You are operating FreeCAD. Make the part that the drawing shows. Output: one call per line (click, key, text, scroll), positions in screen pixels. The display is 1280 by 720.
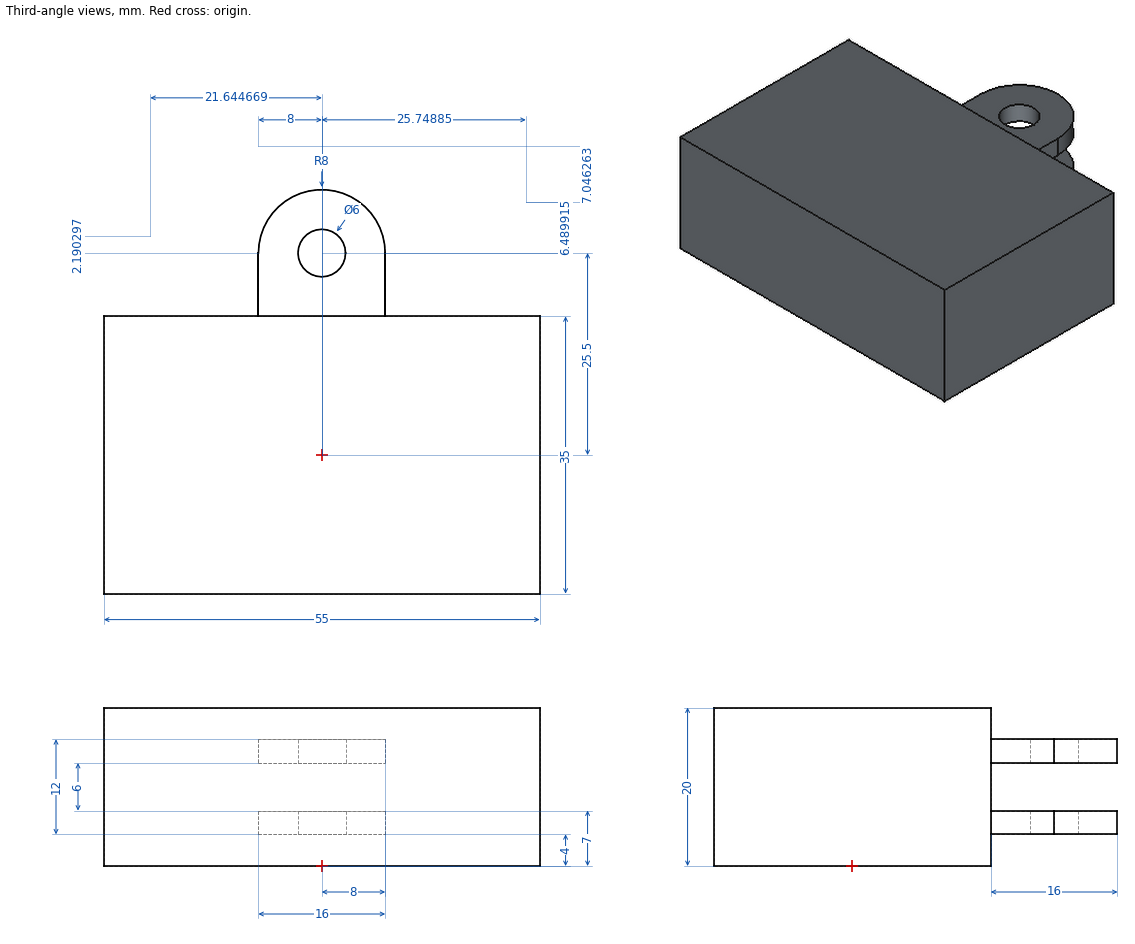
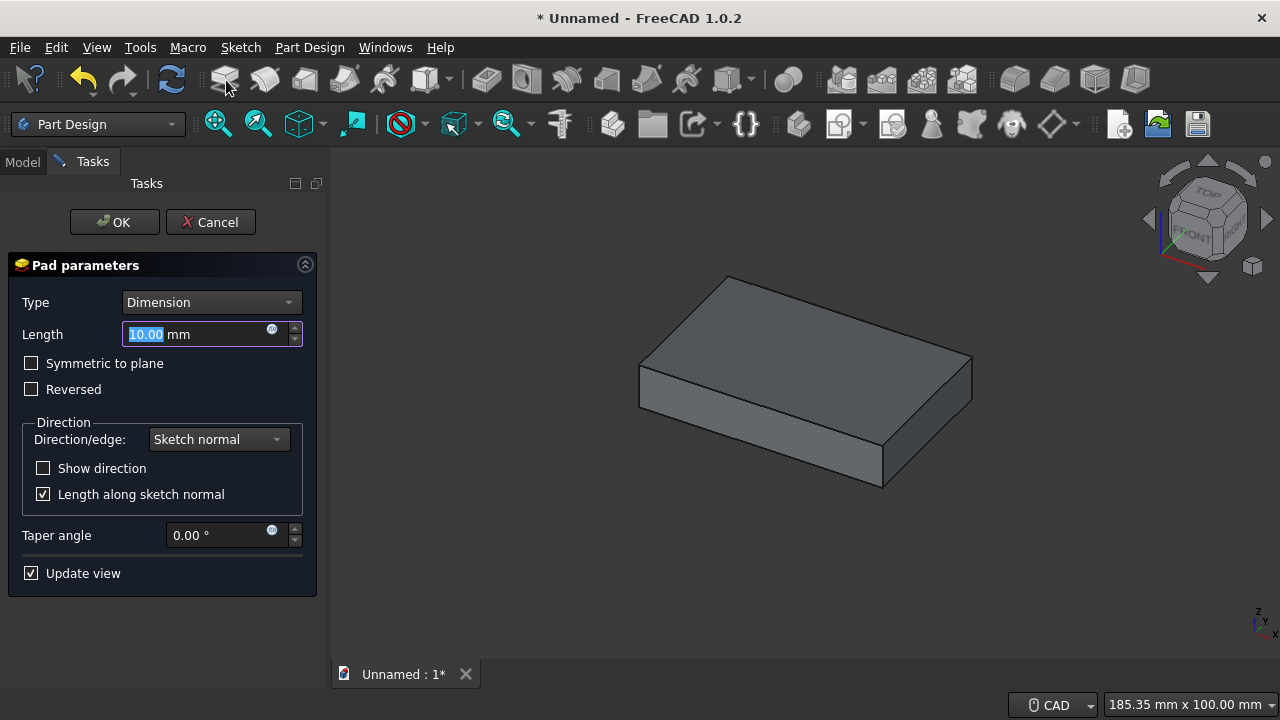
text(20)
key(Tab)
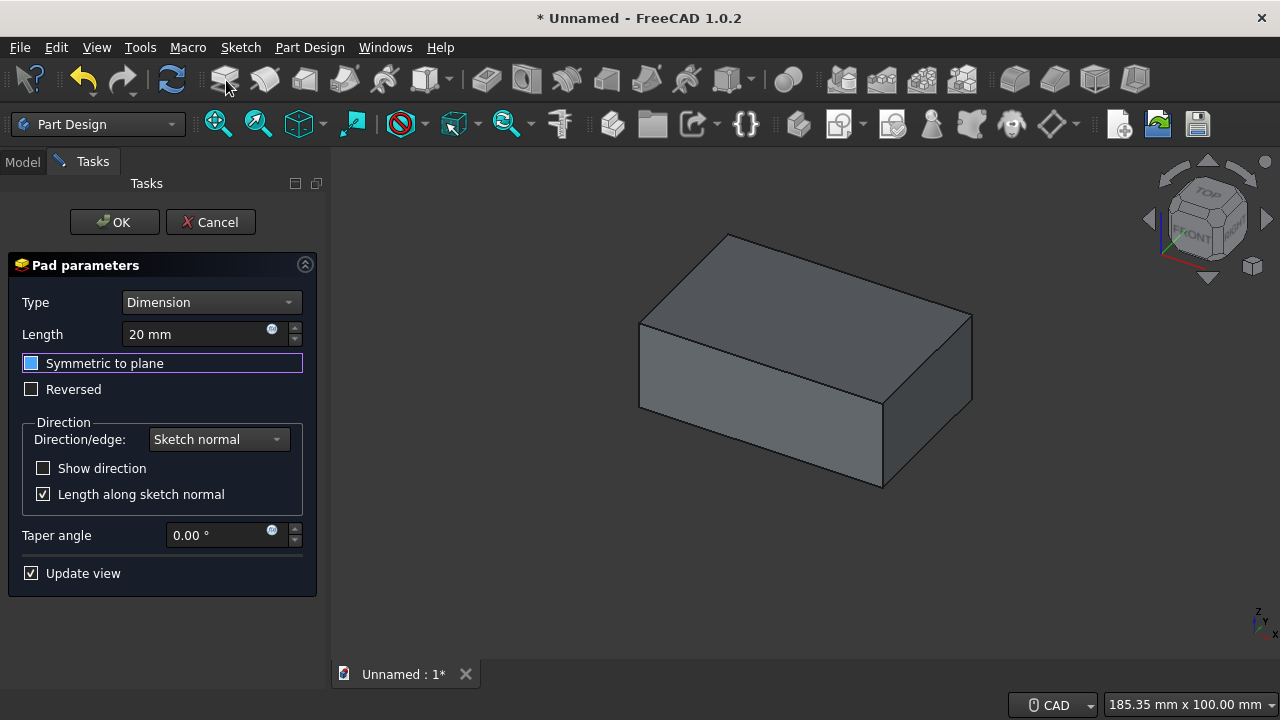
click(115, 222)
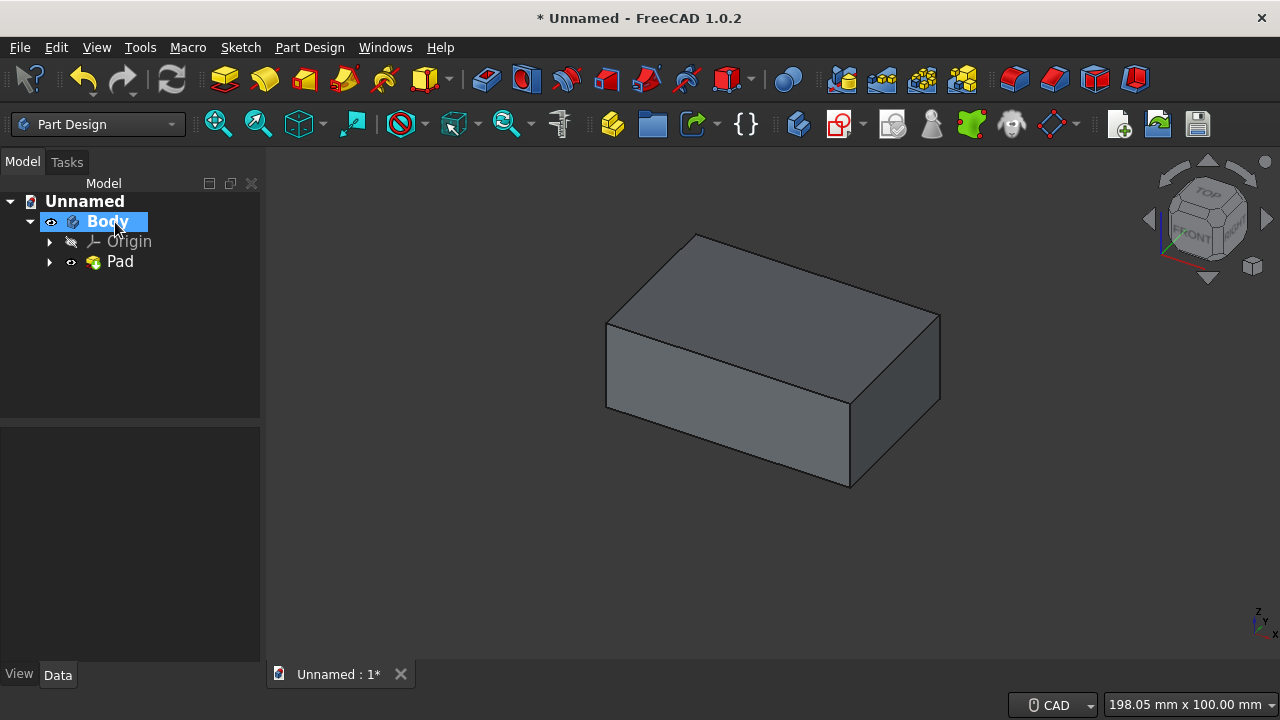
key(4)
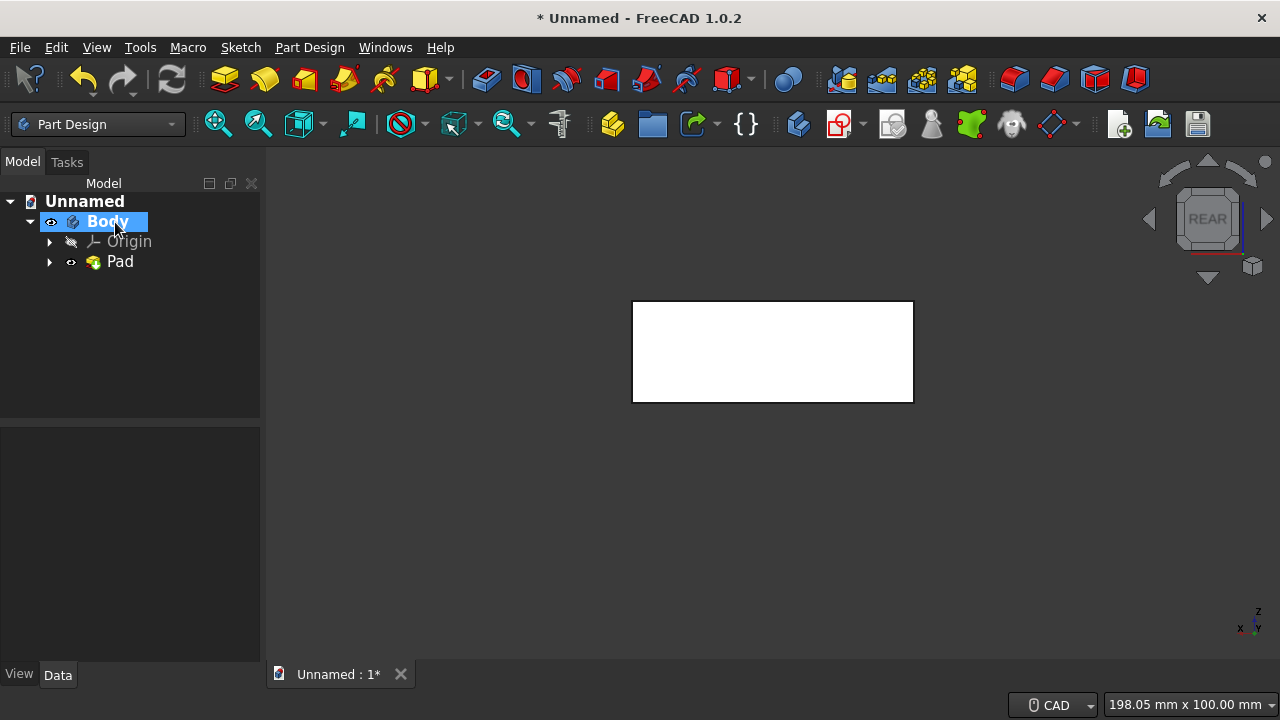
click(220, 124)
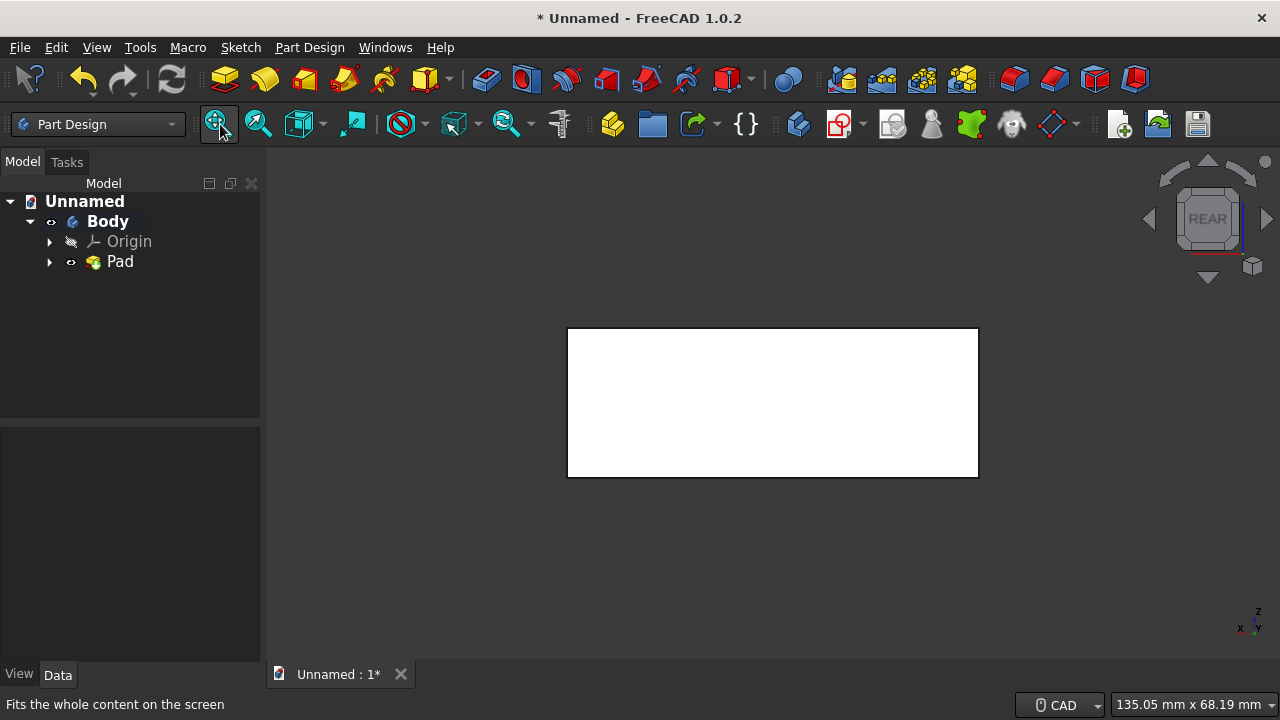
click(655, 402)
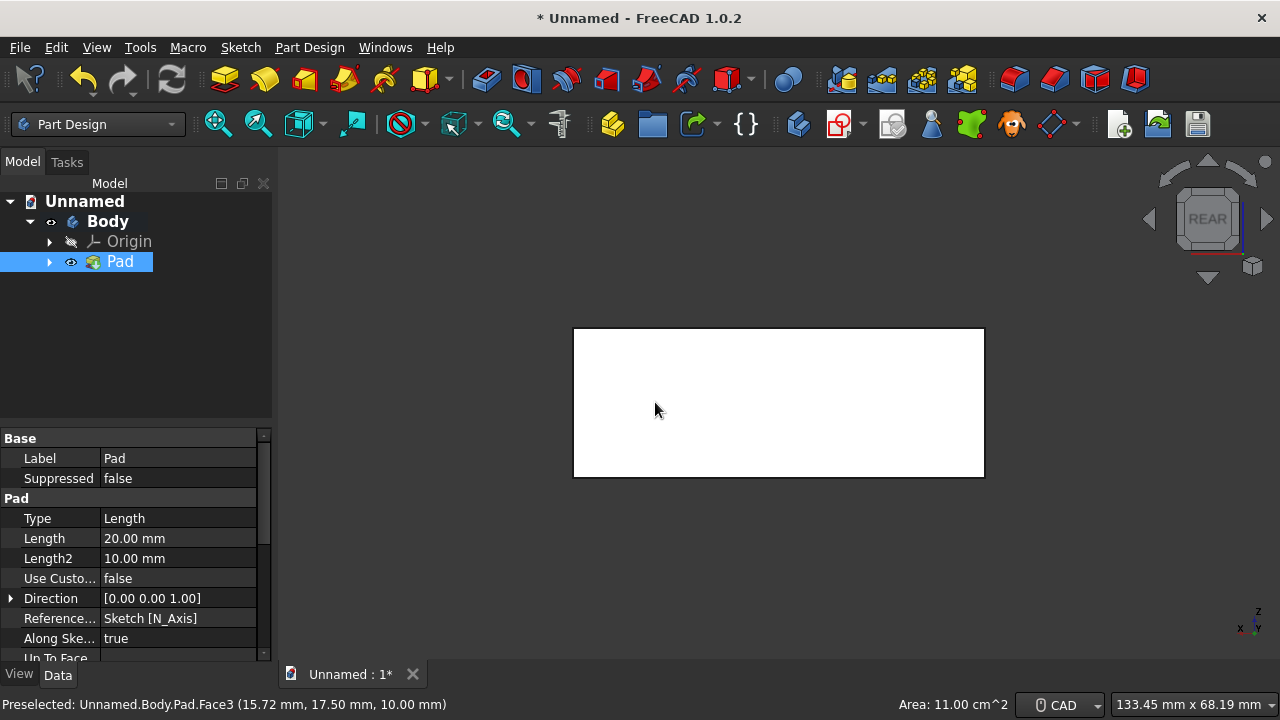
click(840, 124)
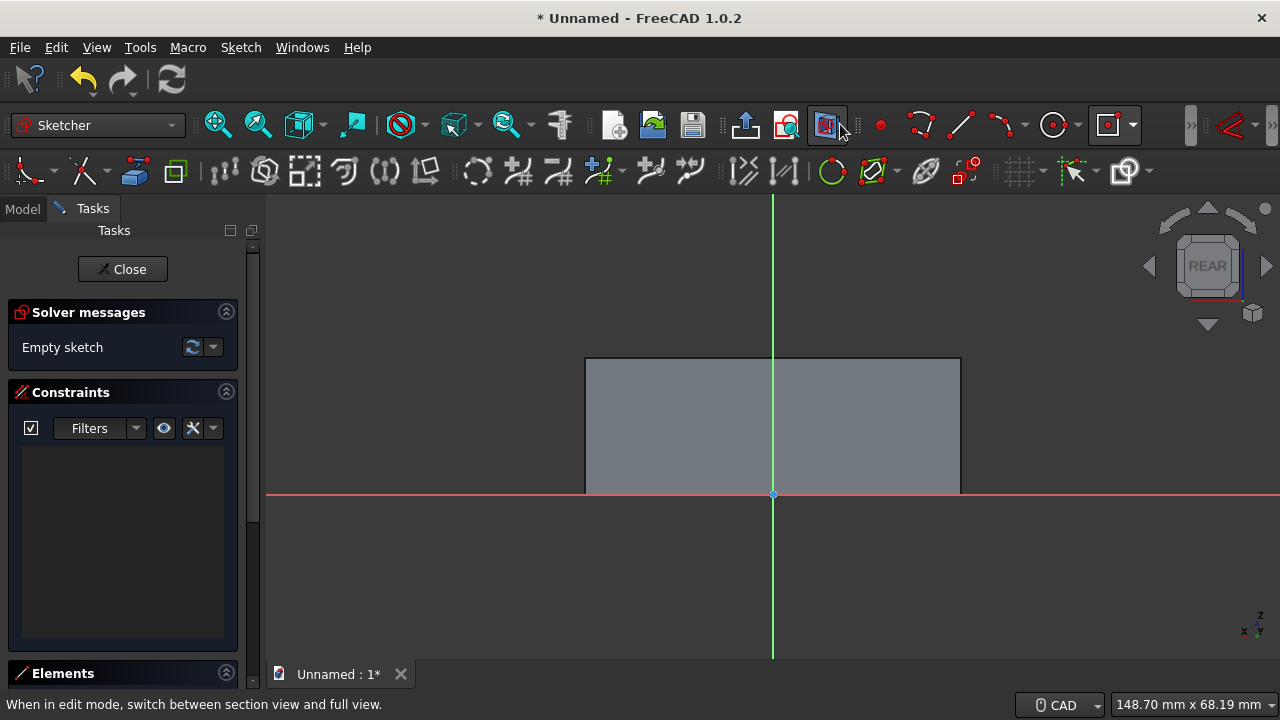
scroll(813, 448, up, 5)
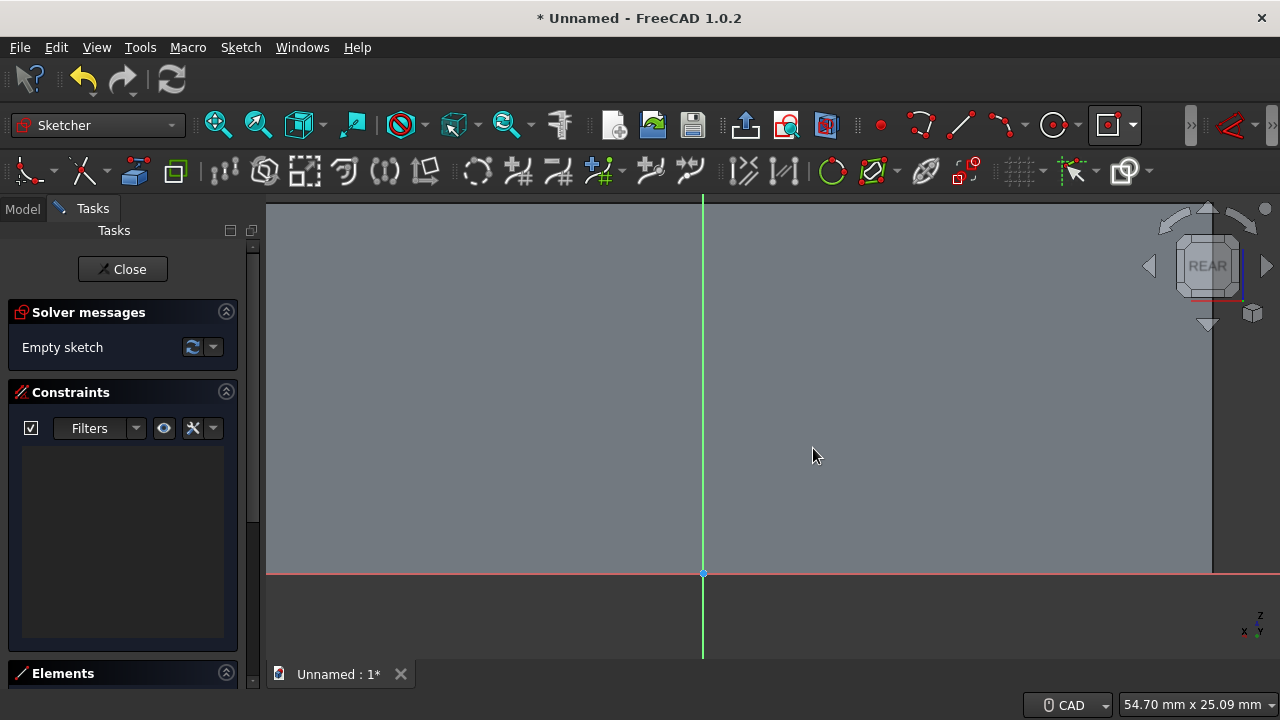
click(1136, 126)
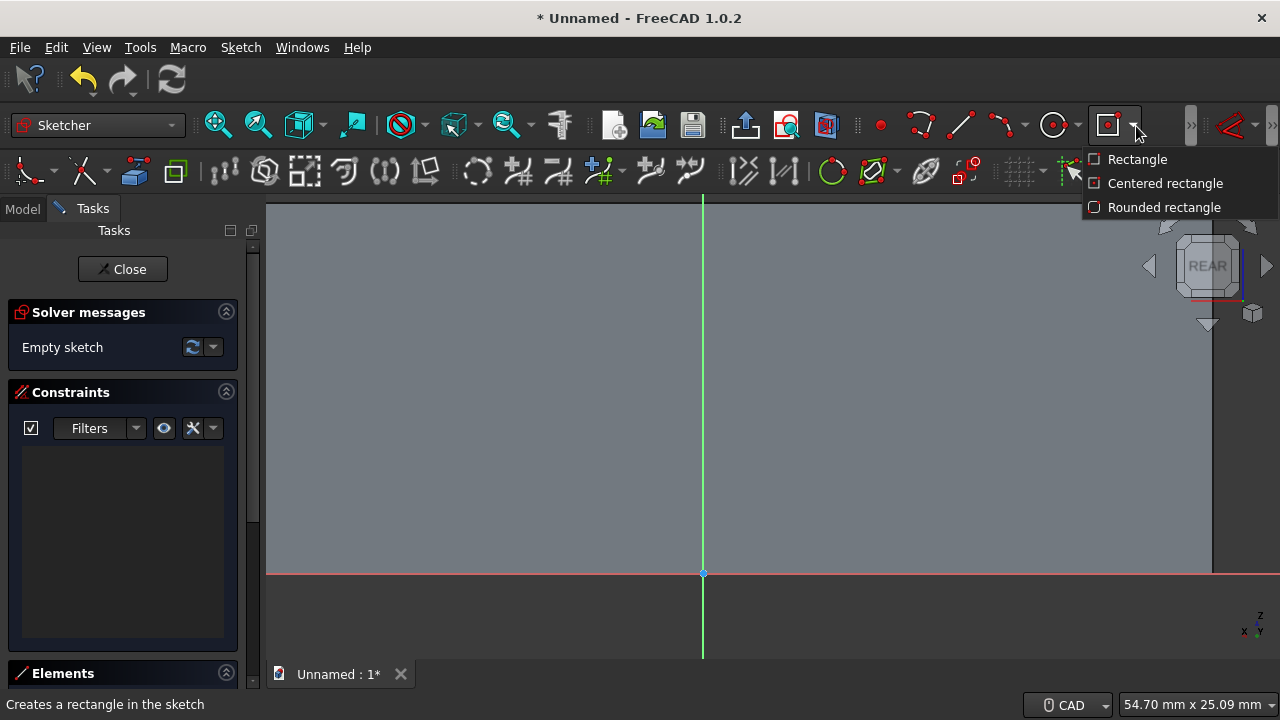
click(1180, 159)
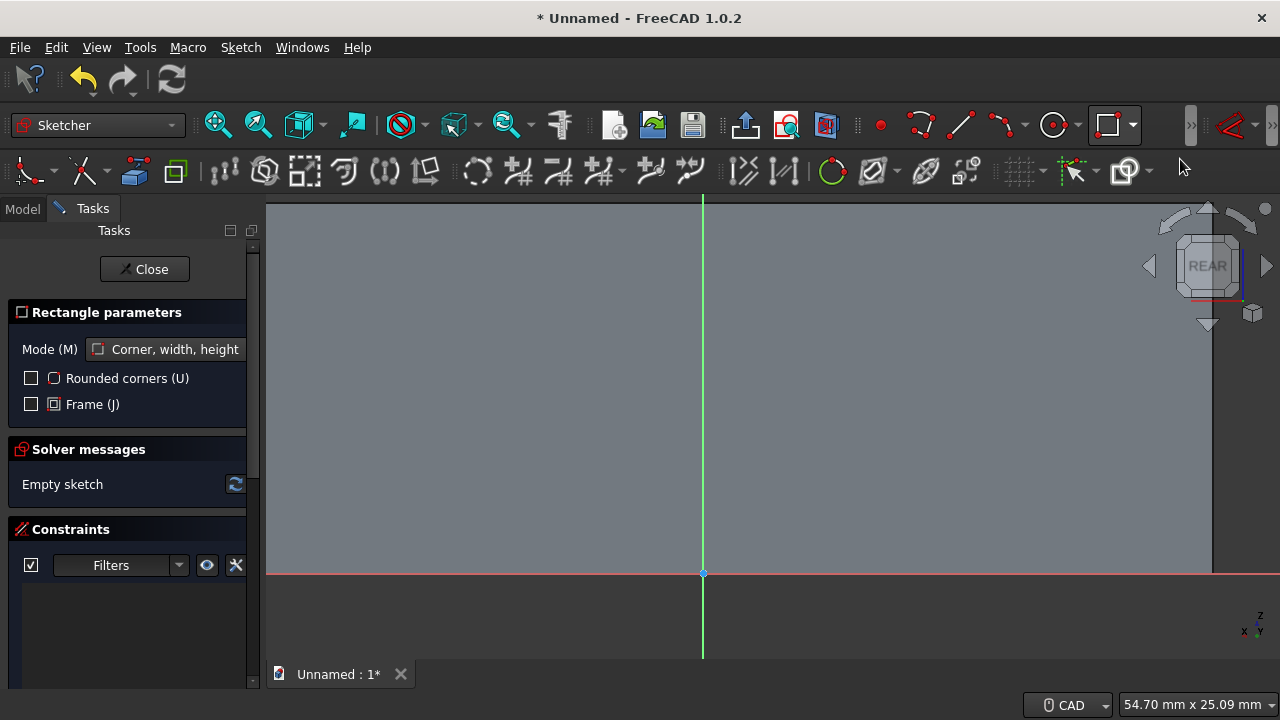
click(555, 277)
move(852, 500)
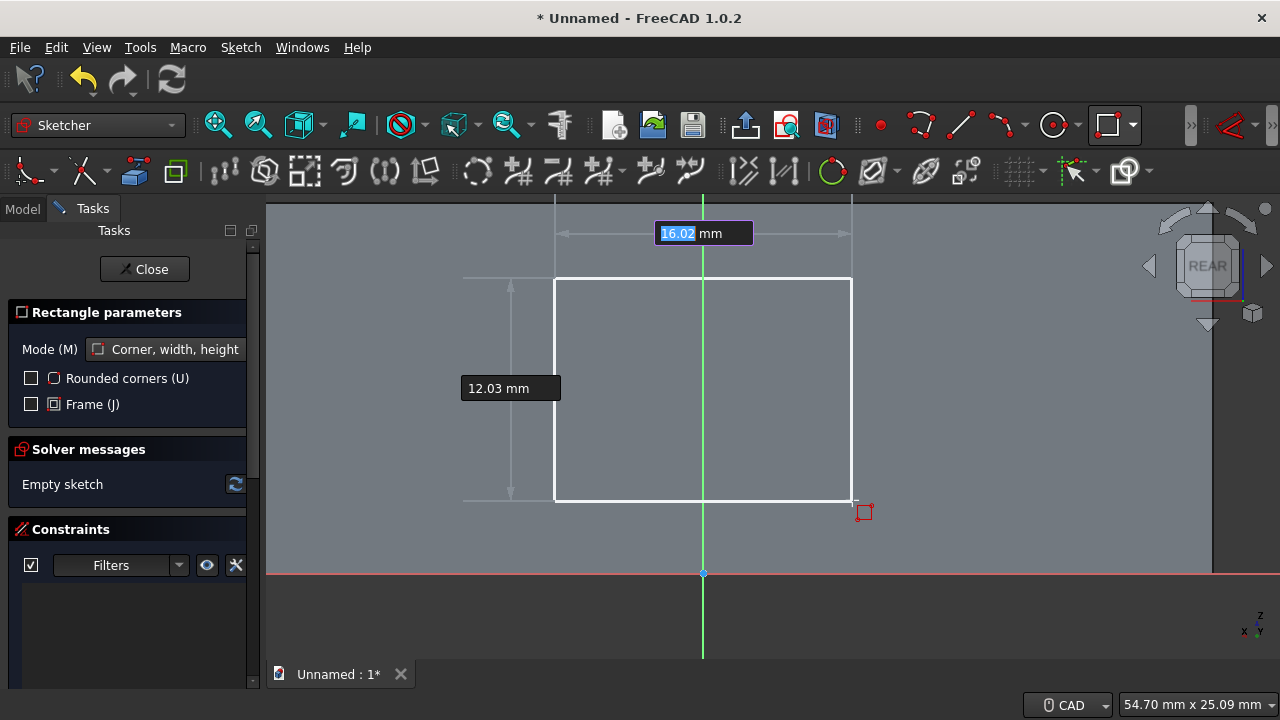
text(16)
key(Tab)
text(12)
key(Return)
key(Escape)